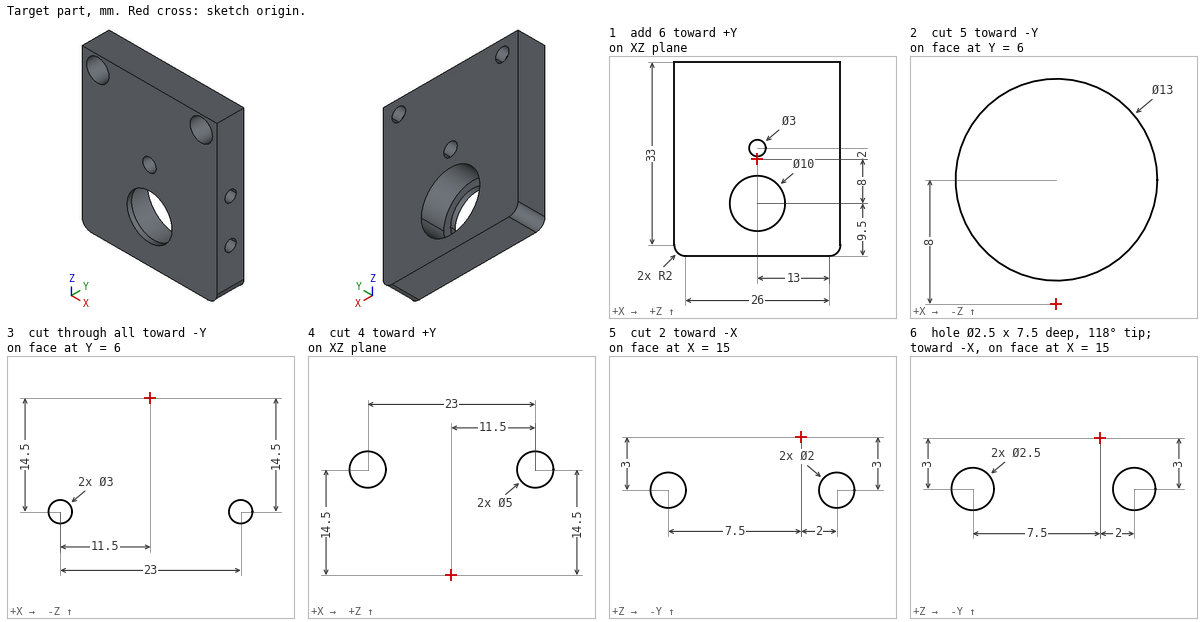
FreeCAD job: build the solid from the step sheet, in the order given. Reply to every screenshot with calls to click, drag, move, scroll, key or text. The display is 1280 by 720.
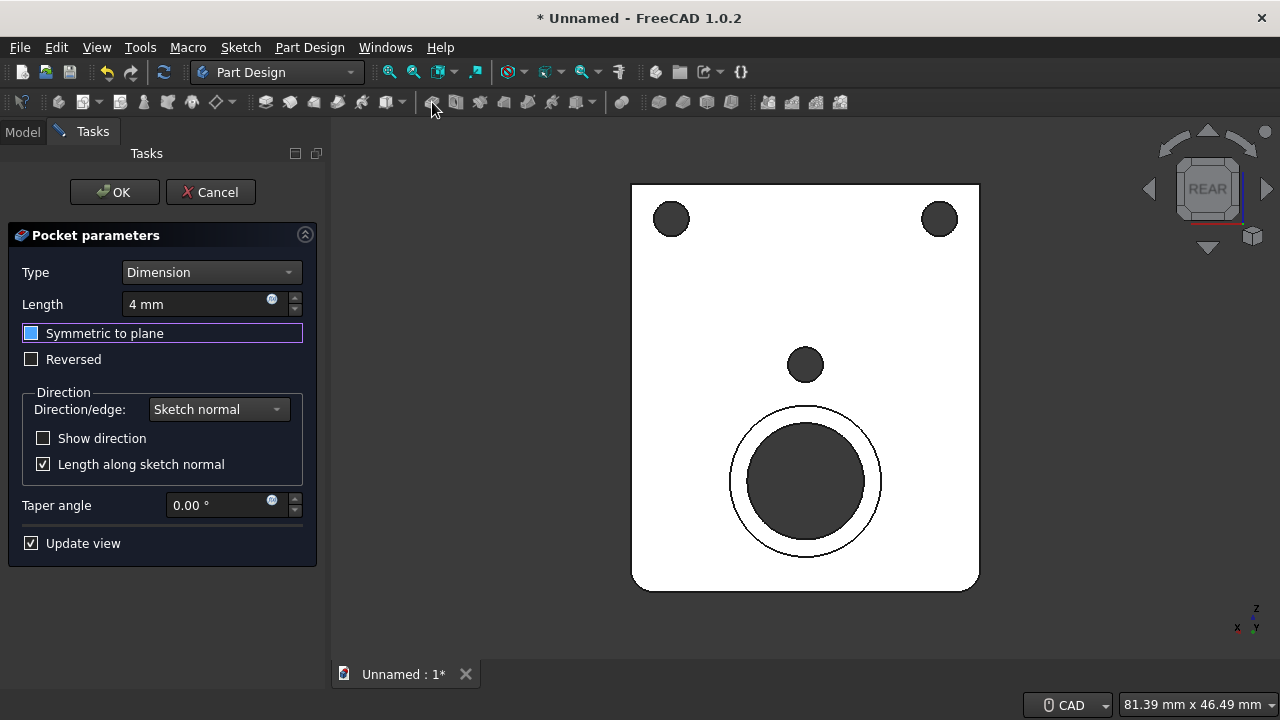
click(115, 192)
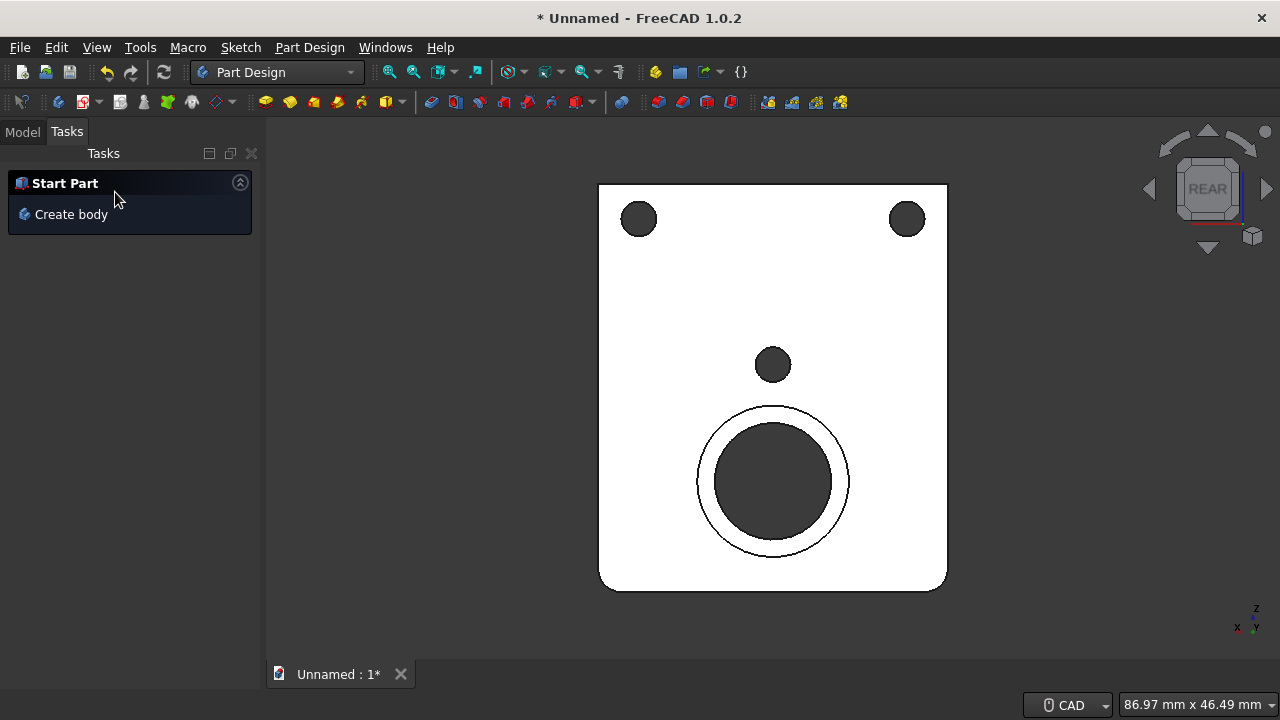
key(0)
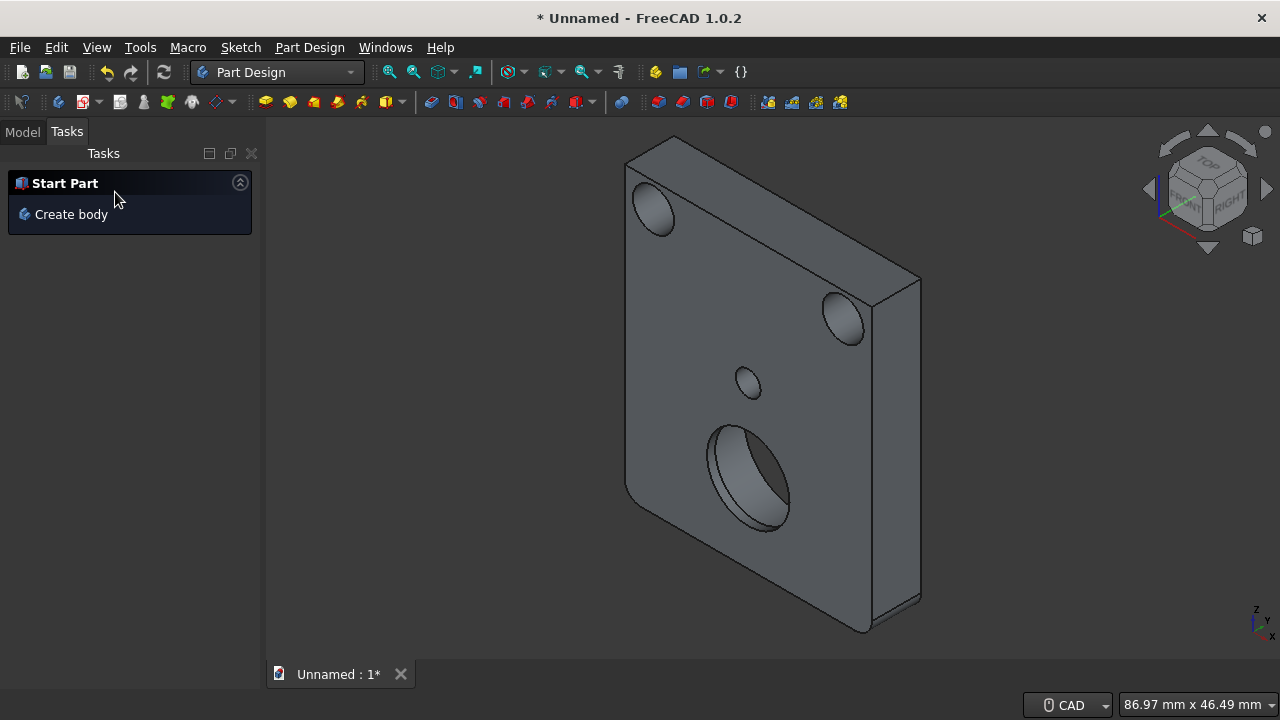
click(897, 494)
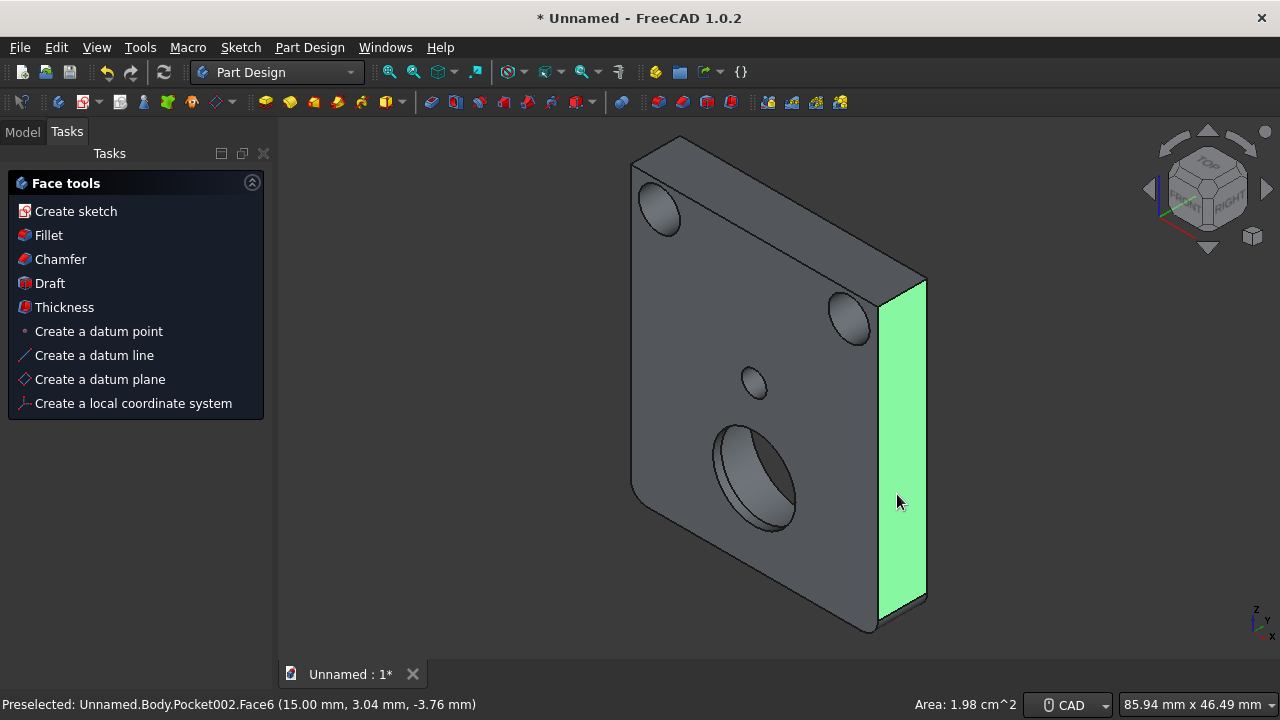
click(84, 102)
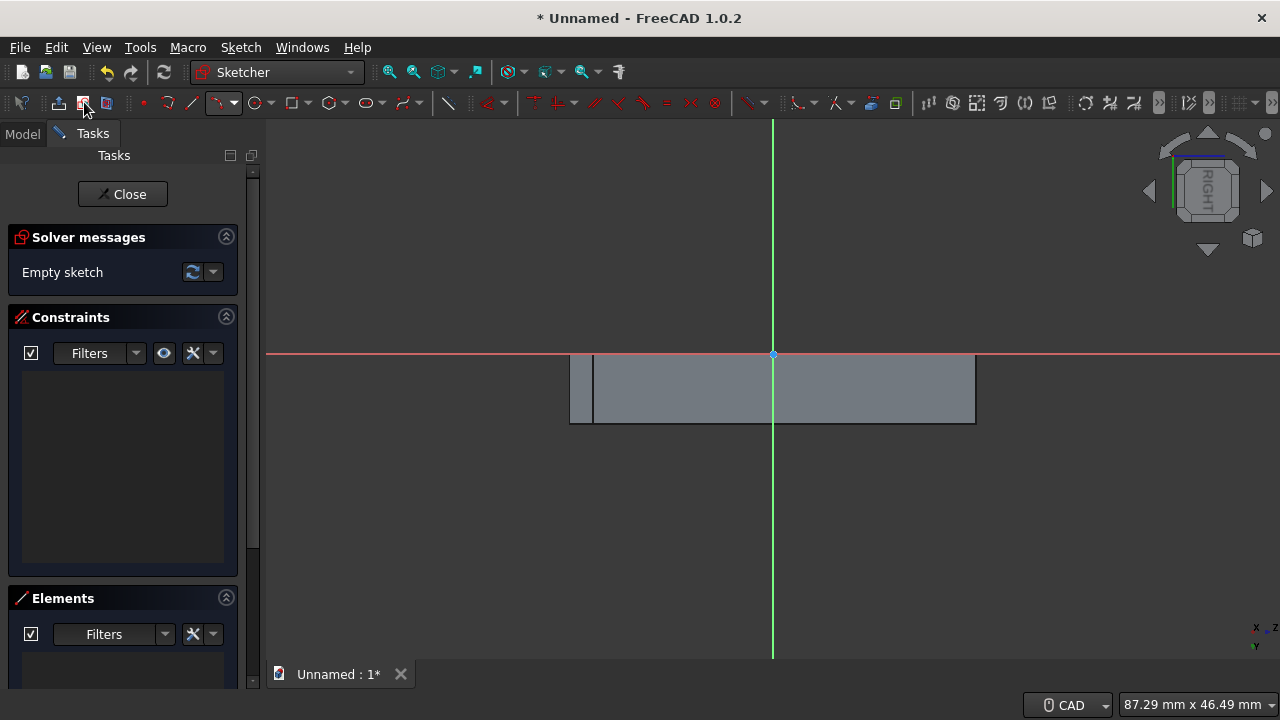
scroll(753, 374, up, 7)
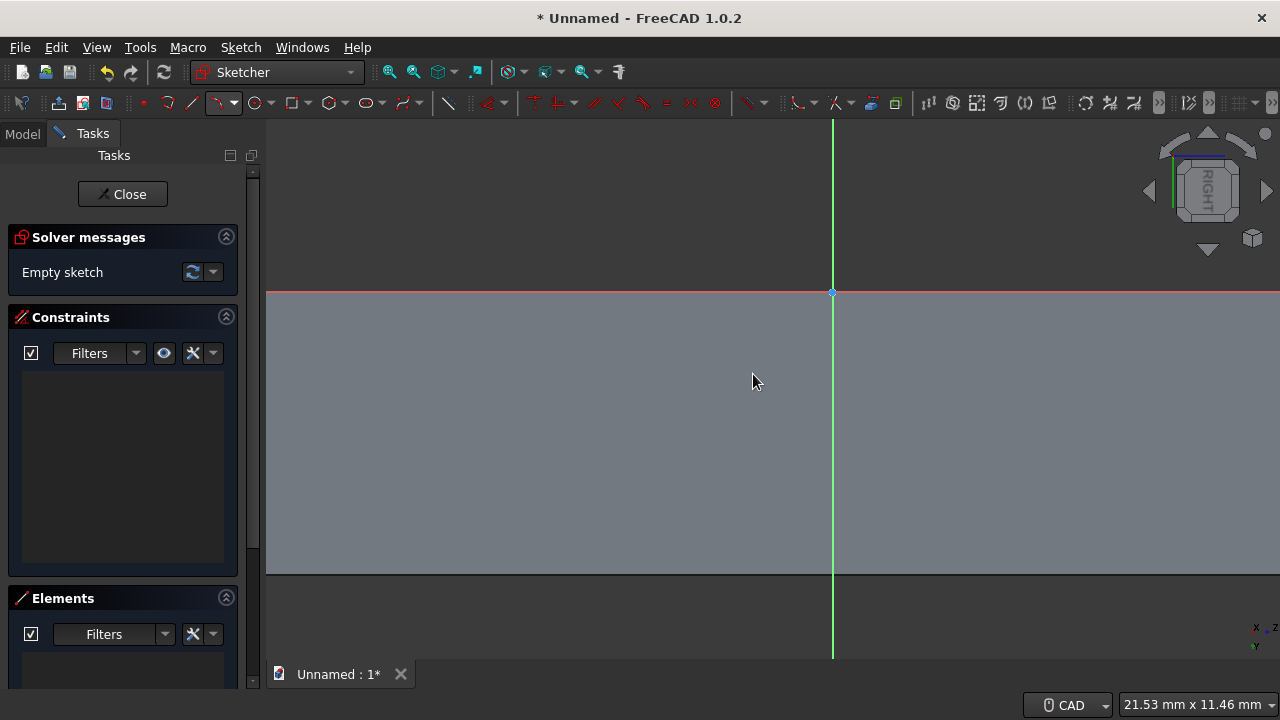
click(256, 104)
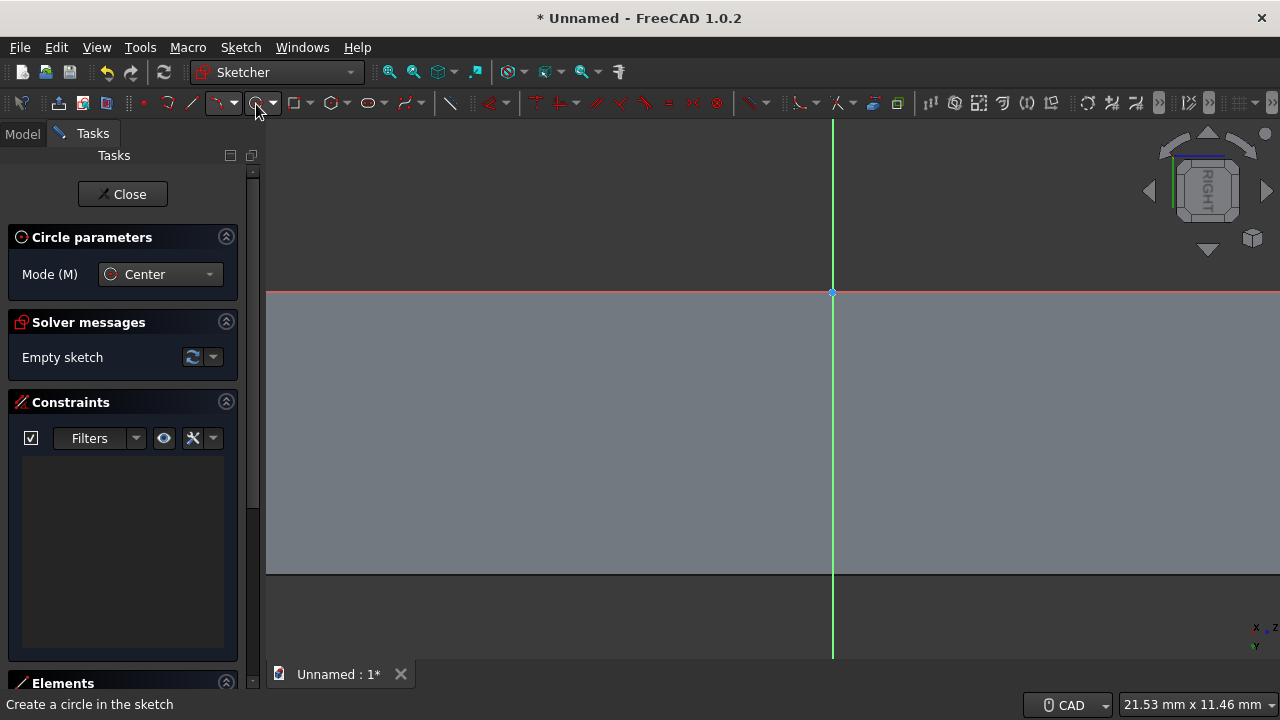
click(927, 433)
click(960, 400)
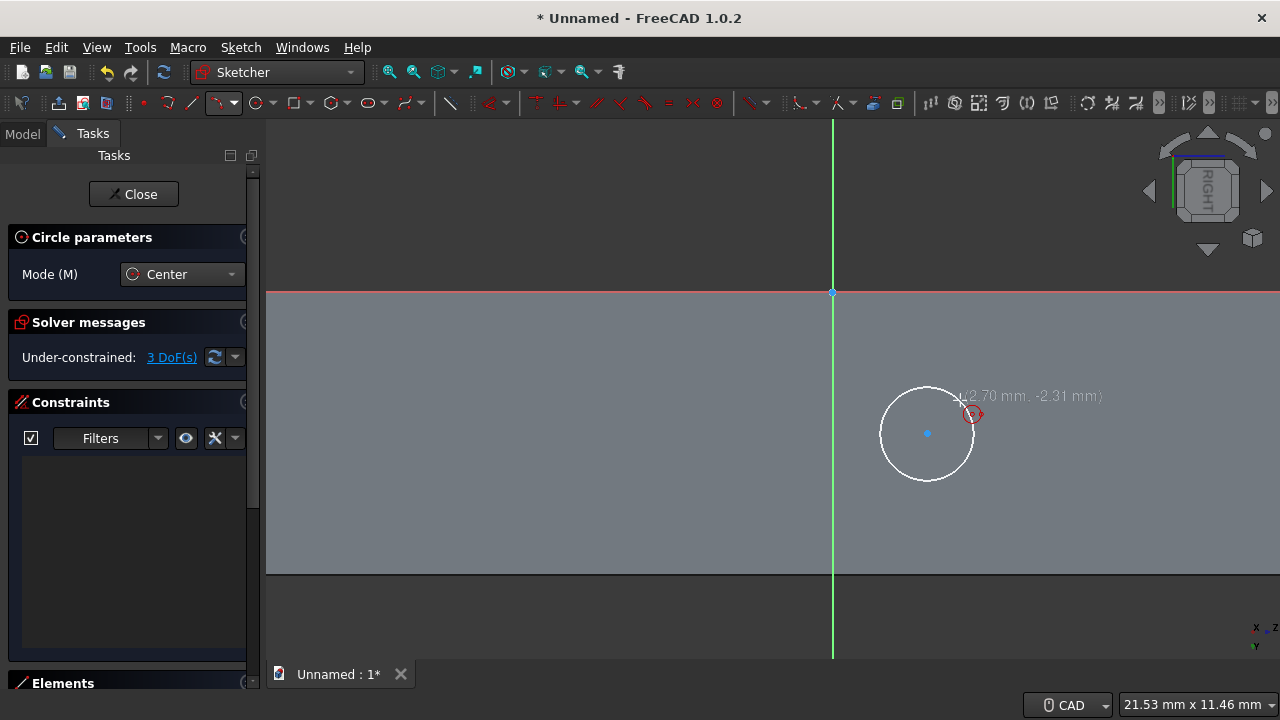
click(479, 433)
click(513, 400)
key(Escape)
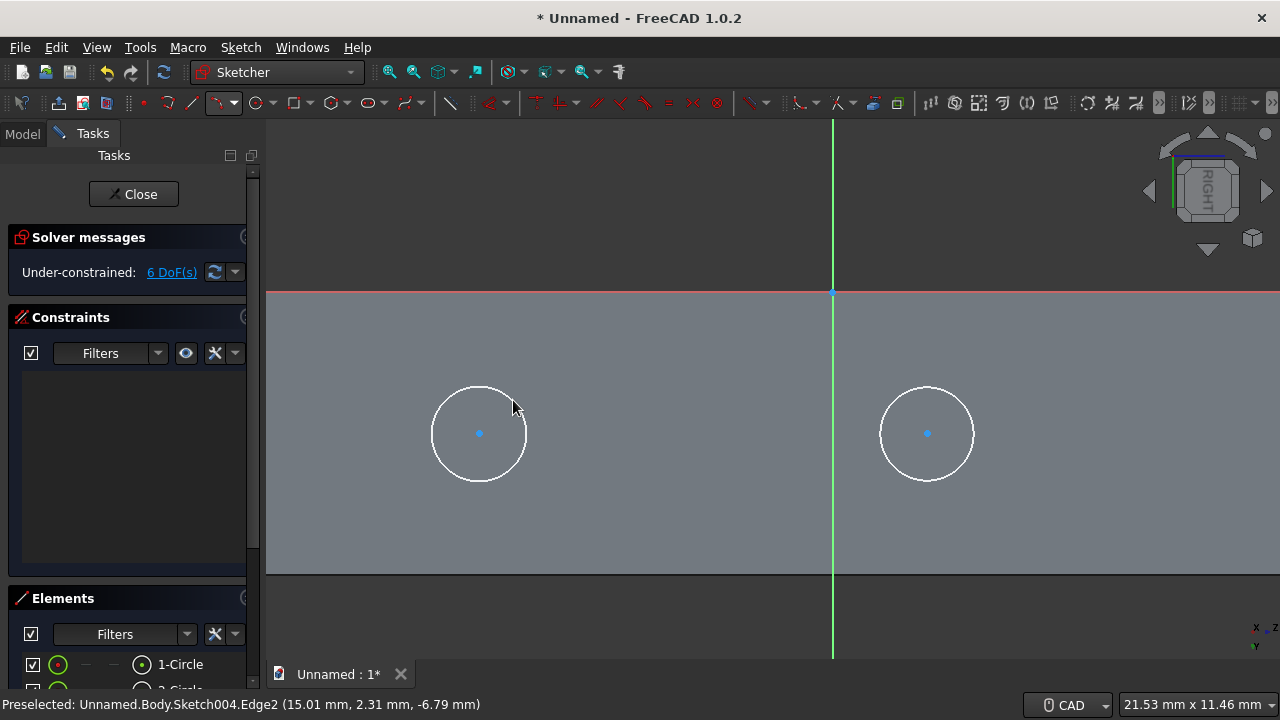
click(960, 401)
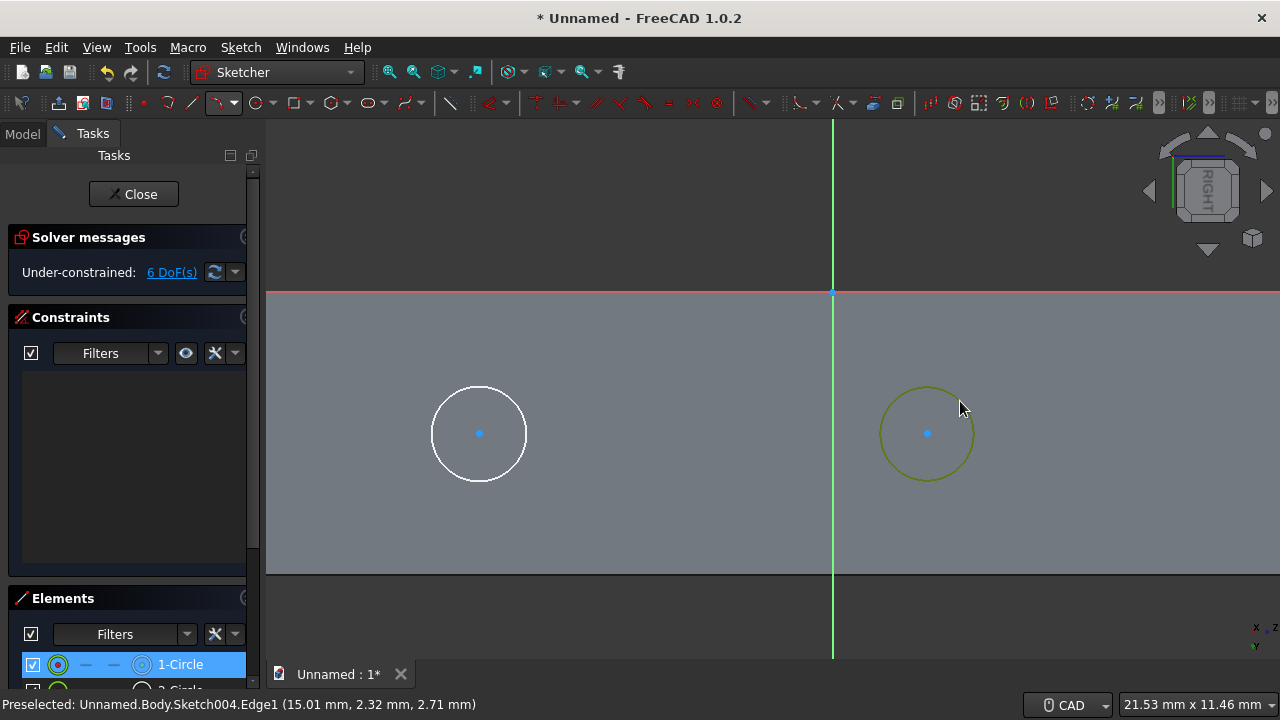
click(512, 400)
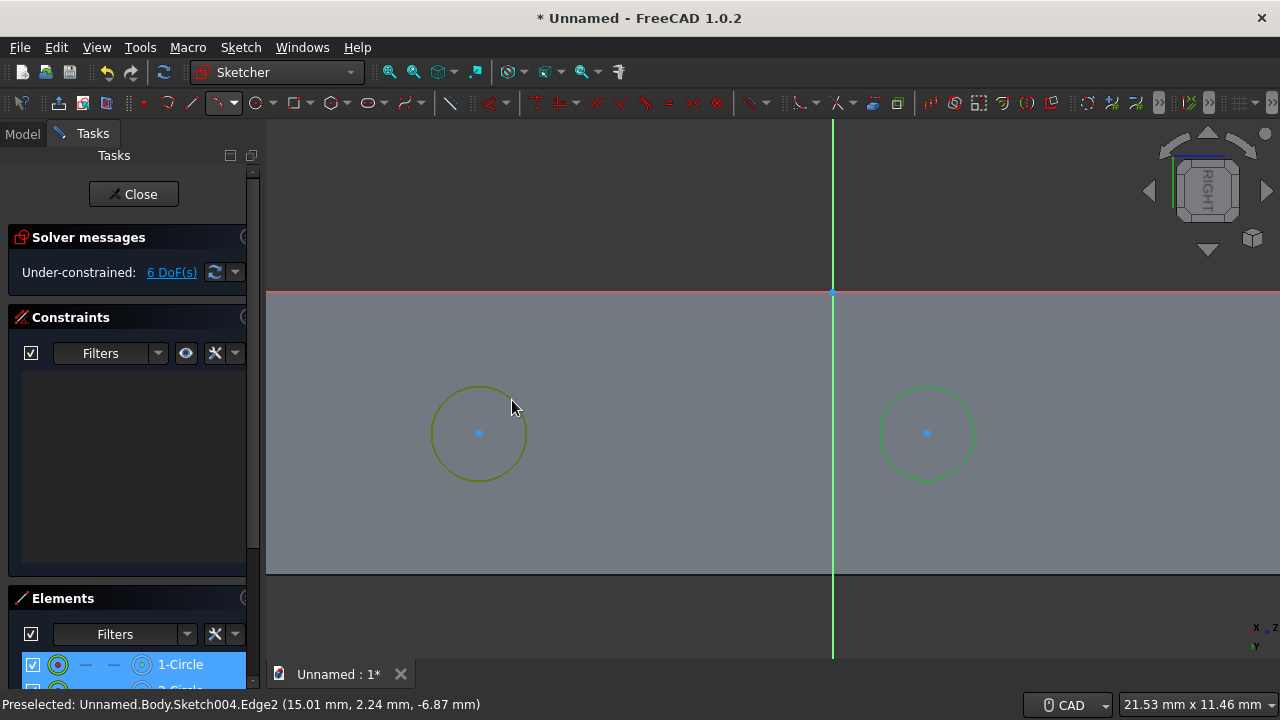
click(670, 104)